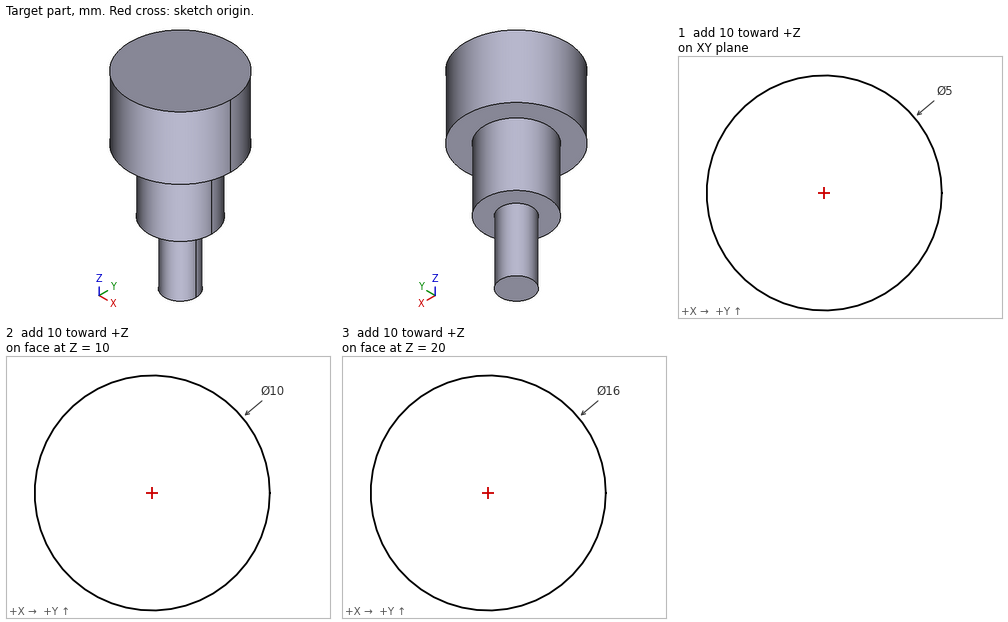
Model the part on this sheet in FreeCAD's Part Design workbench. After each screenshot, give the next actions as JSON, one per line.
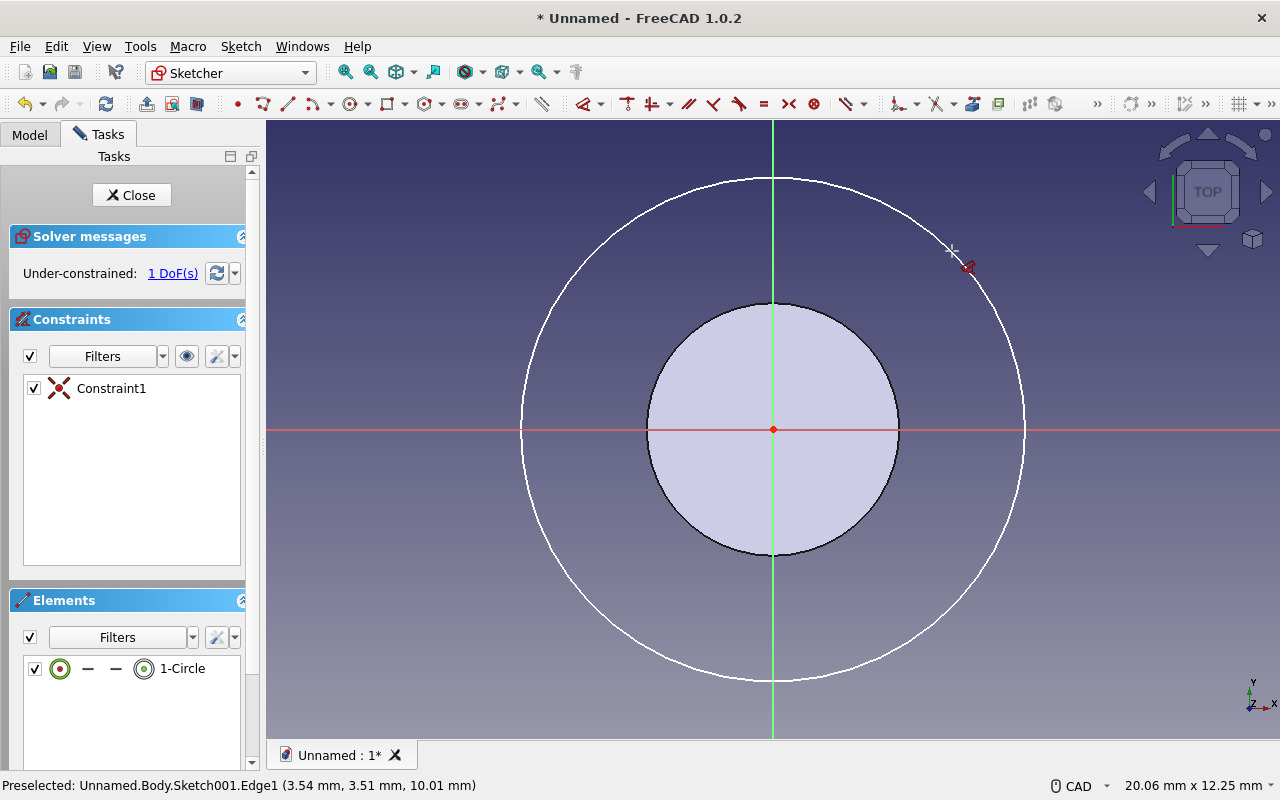
{"action": "left_click", "coordinate": [951, 251]}
{"action": "left_click", "coordinate": [974, 228]}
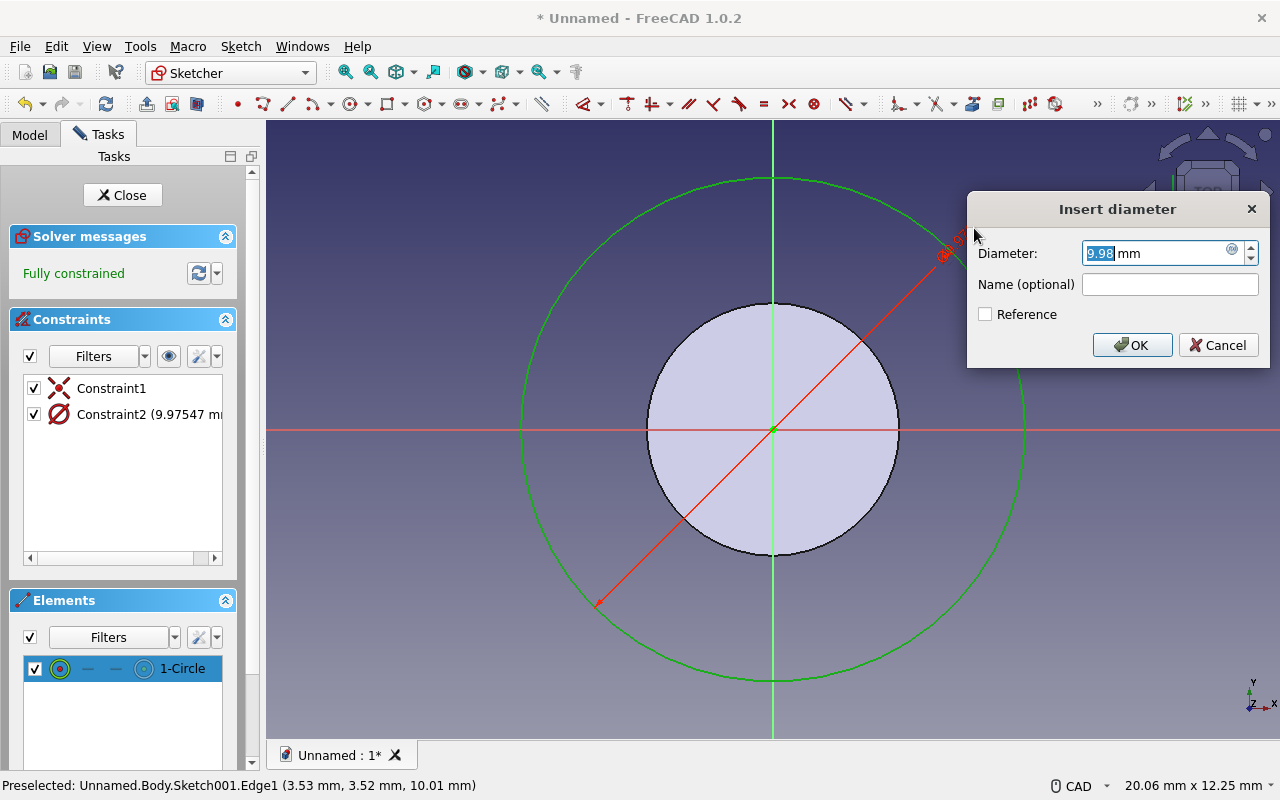
{"action": "type", "text": "10"}
{"action": "key", "text": "Return"}
{"action": "key", "text": "Escape"}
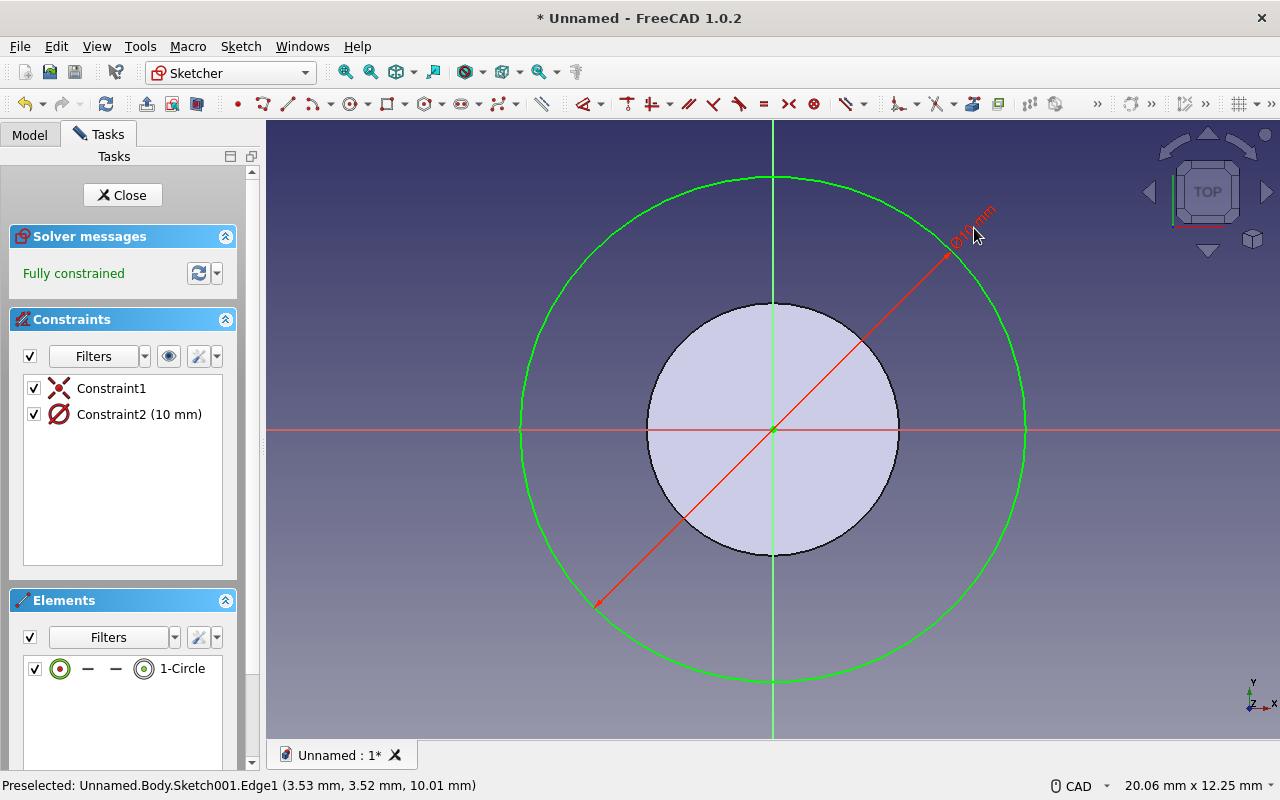
{"action": "left_click", "coordinate": [123, 195]}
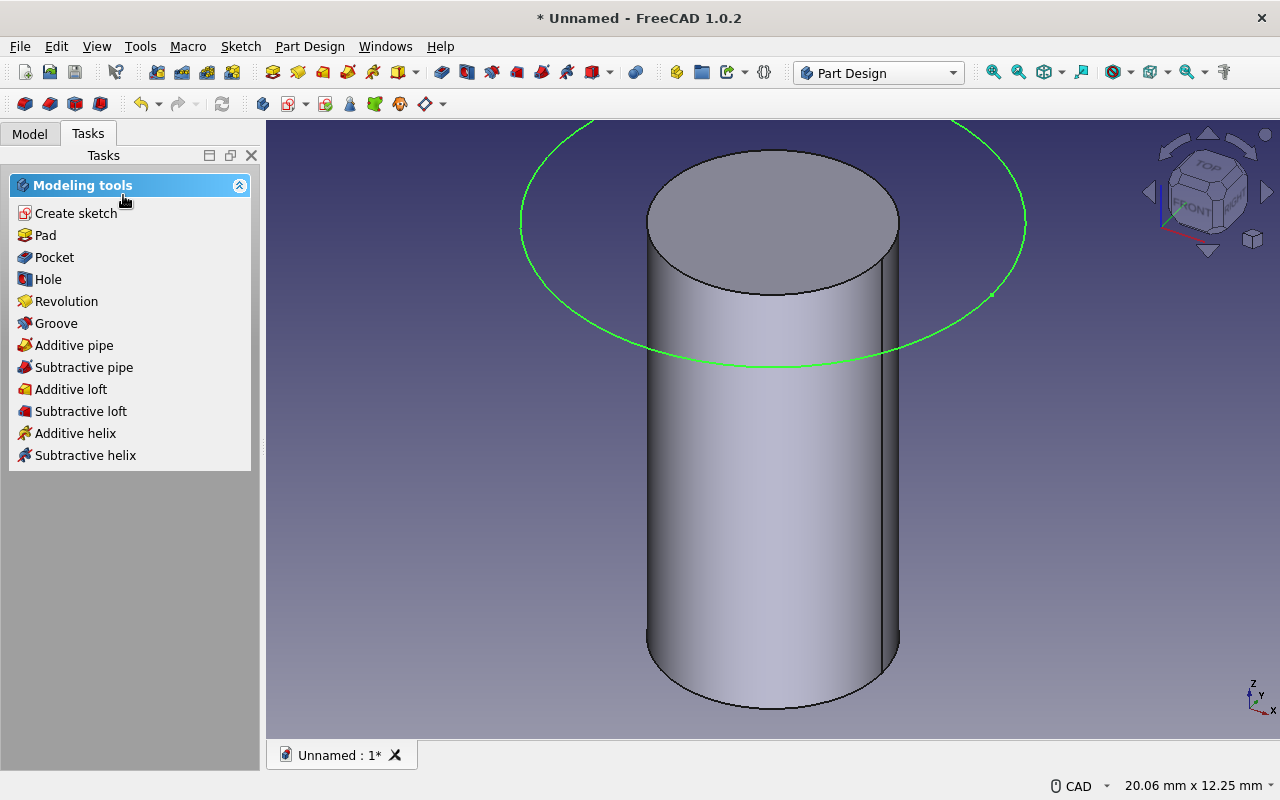
{"action": "left_click", "coordinate": [273, 72]}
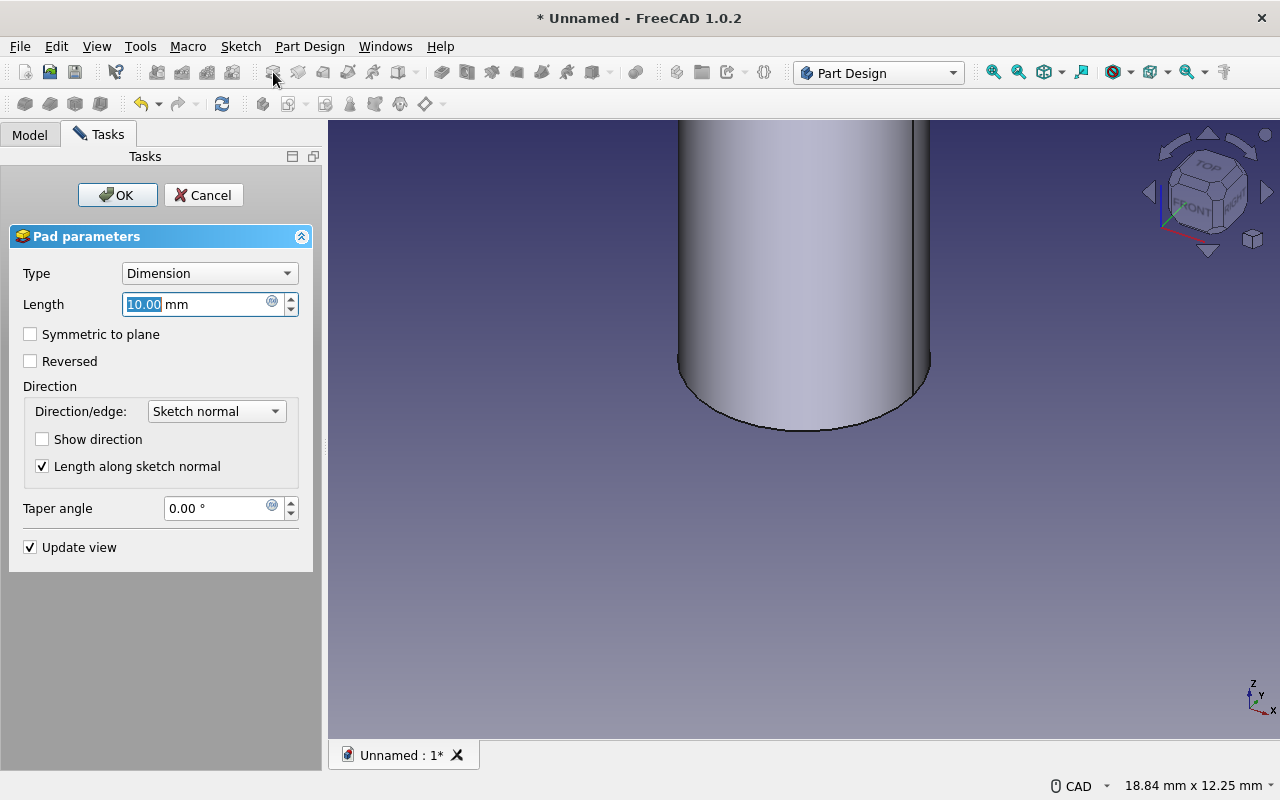
{"action": "type", "text": "10"}
{"action": "key", "text": "Tab"}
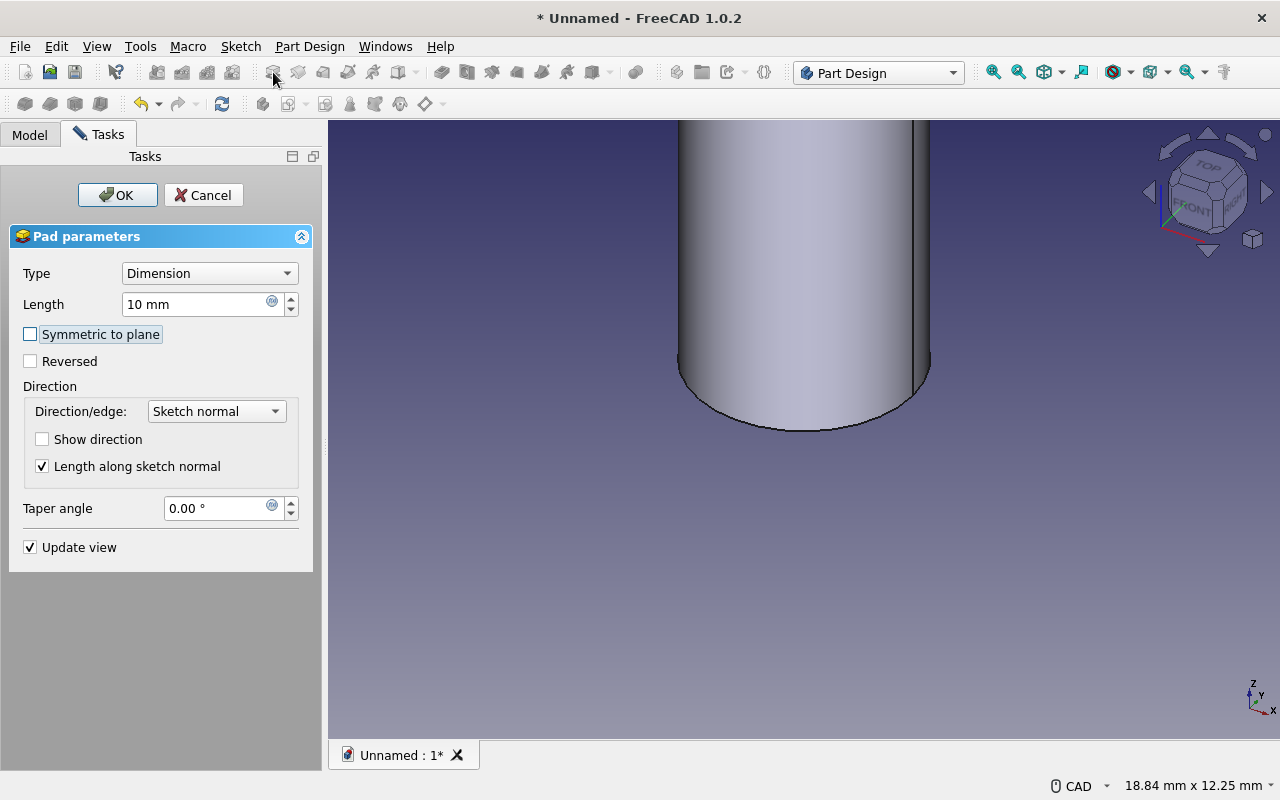
{"action": "left_click", "coordinate": [118, 195]}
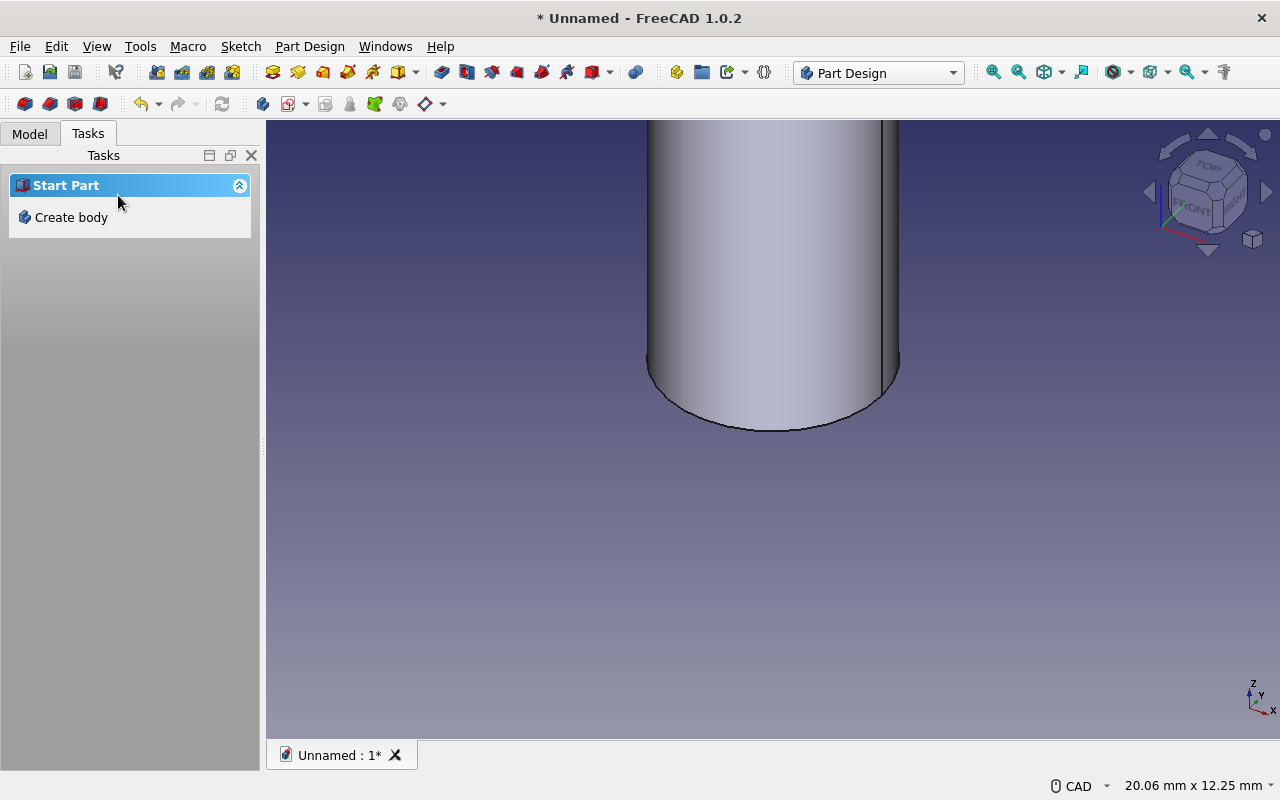
{"action": "left_click", "coordinate": [994, 72]}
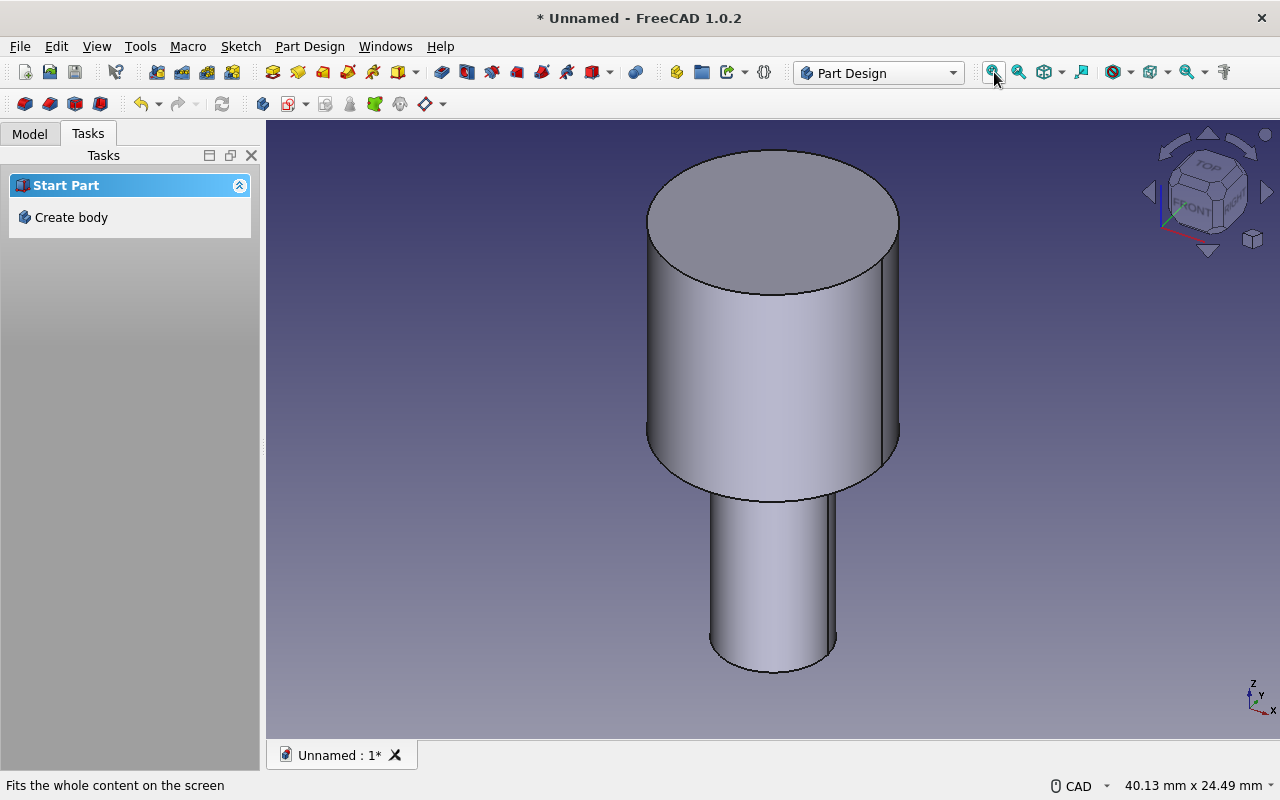
{"action": "left_click", "coordinate": [773, 221]}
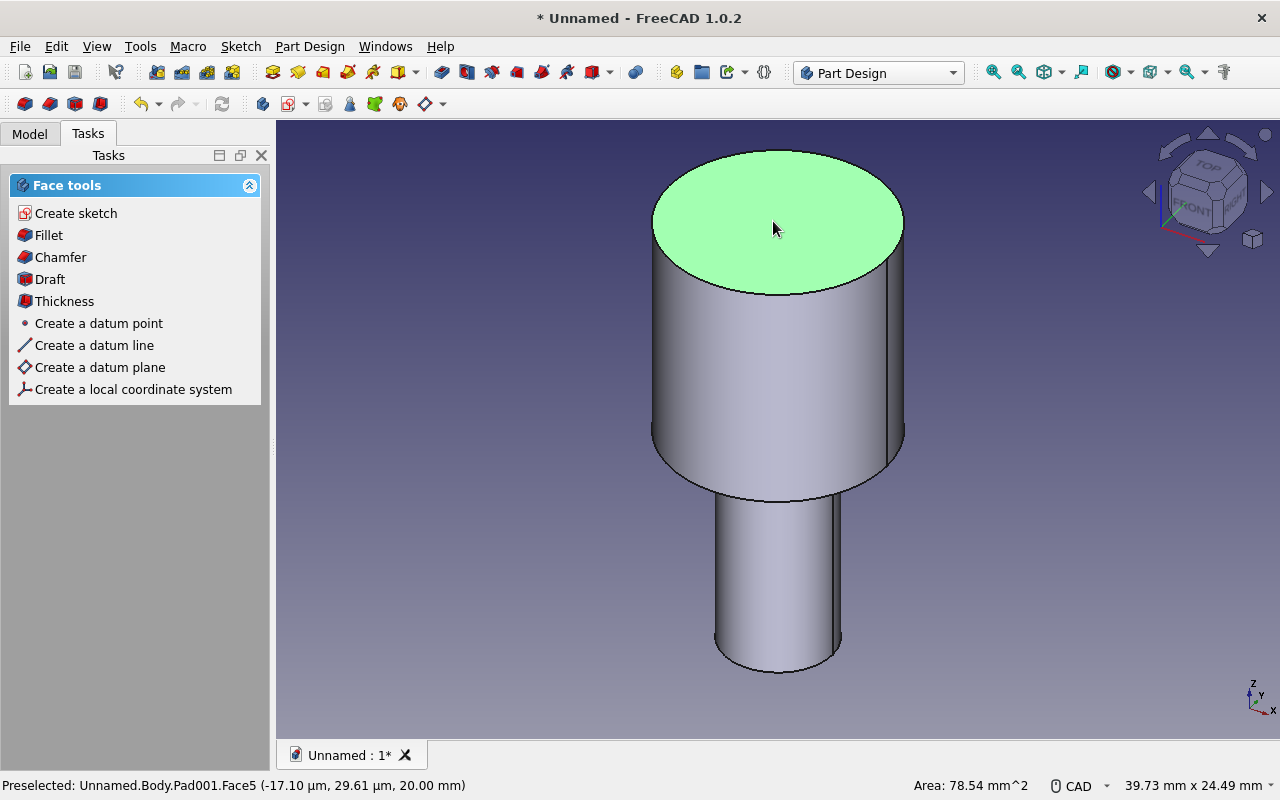
{"action": "left_click", "coordinate": [288, 104]}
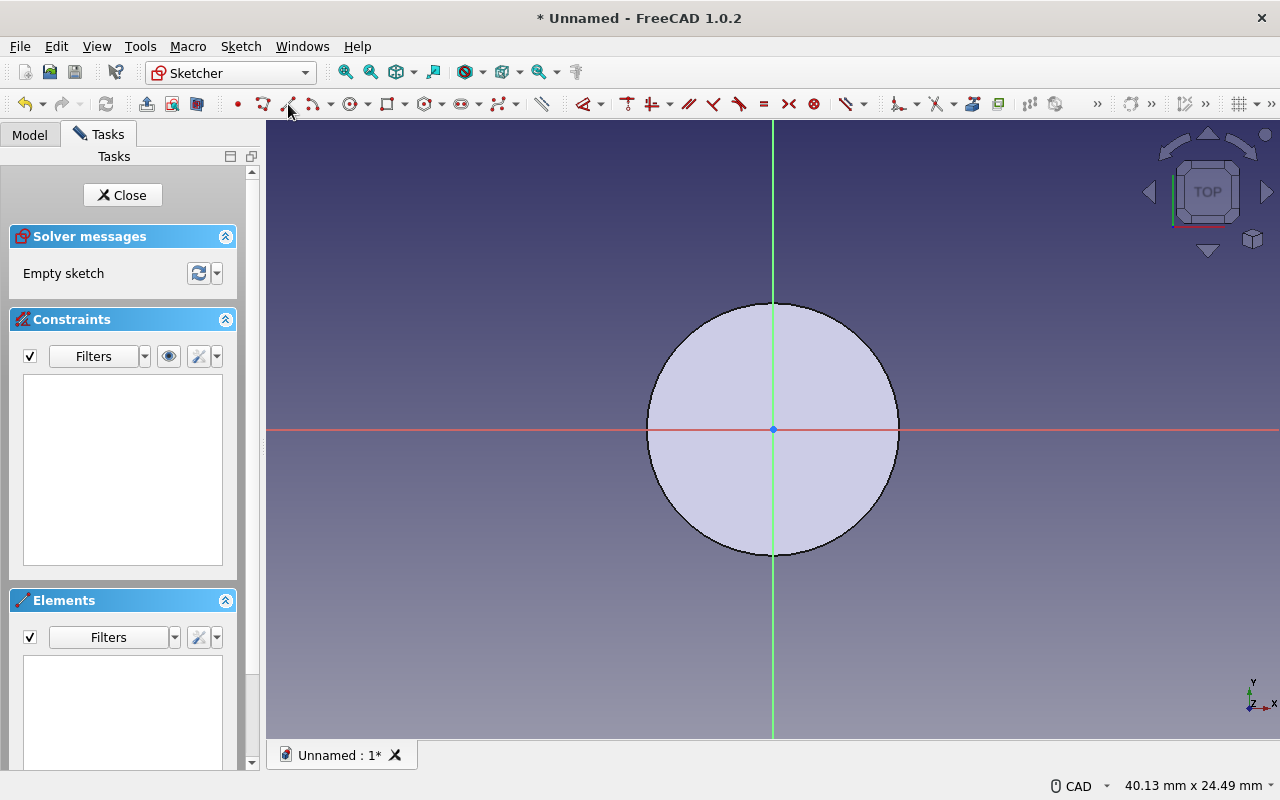
{"action": "left_click", "coordinate": [350, 104]}